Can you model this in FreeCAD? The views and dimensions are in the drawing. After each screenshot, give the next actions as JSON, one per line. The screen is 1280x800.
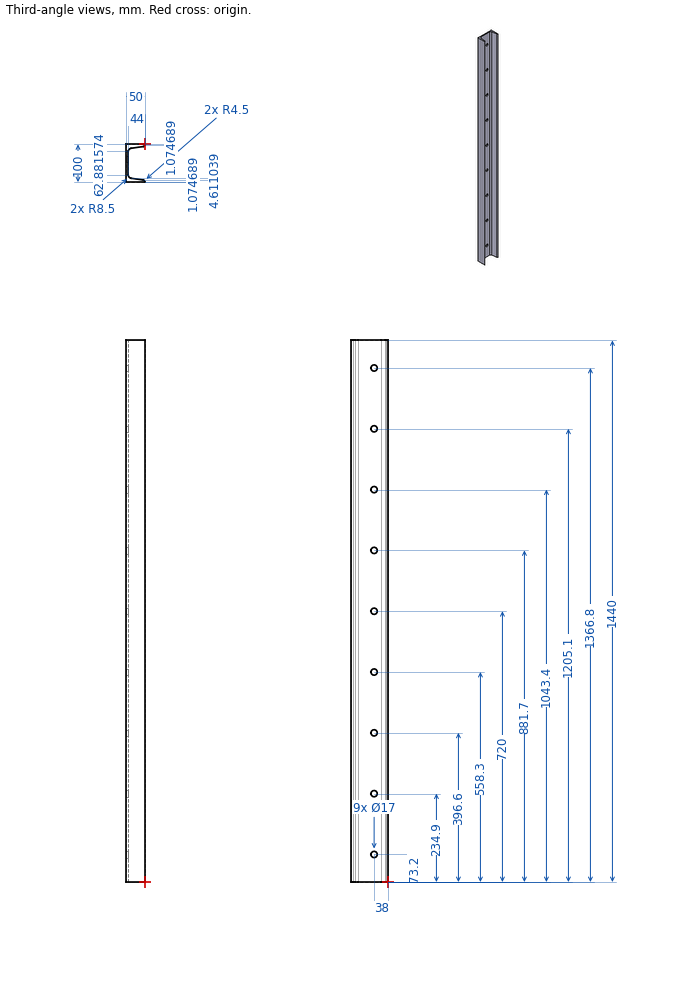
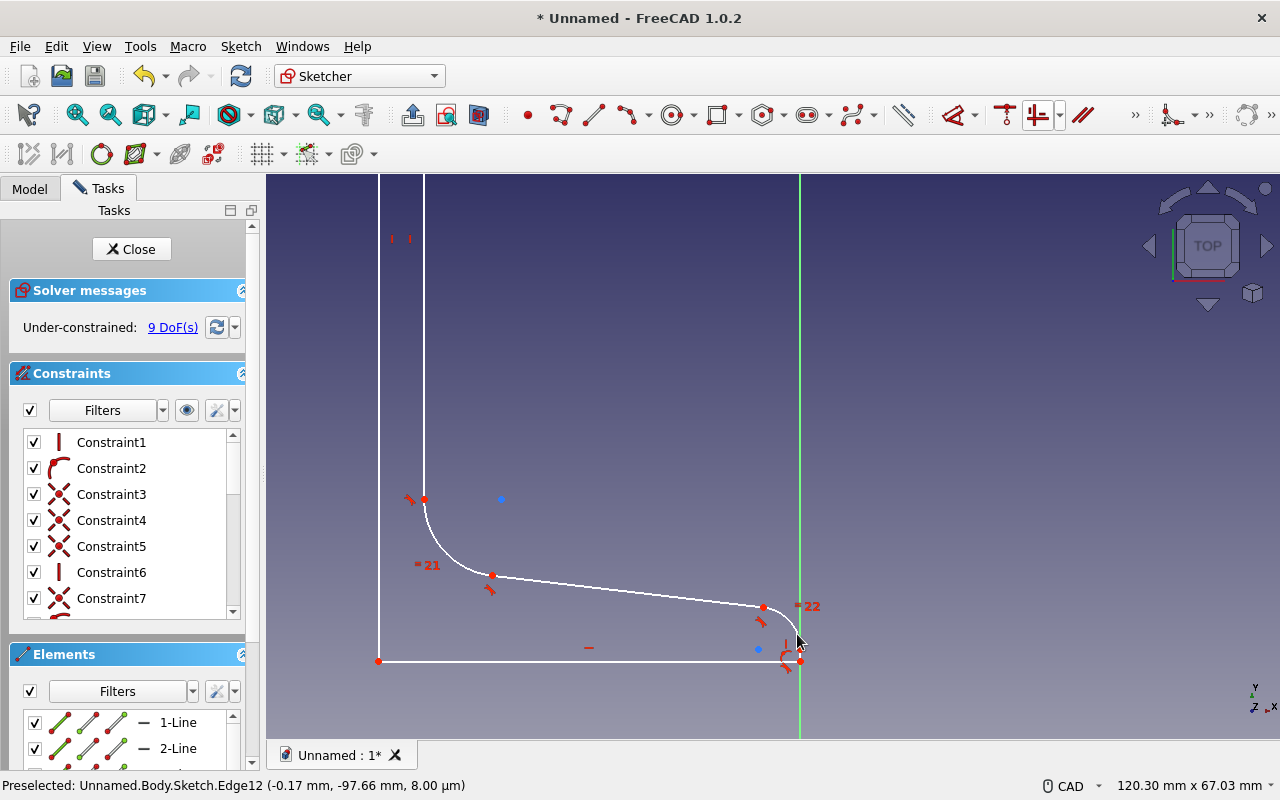
{"action": "left_click", "coordinate": [431, 532]}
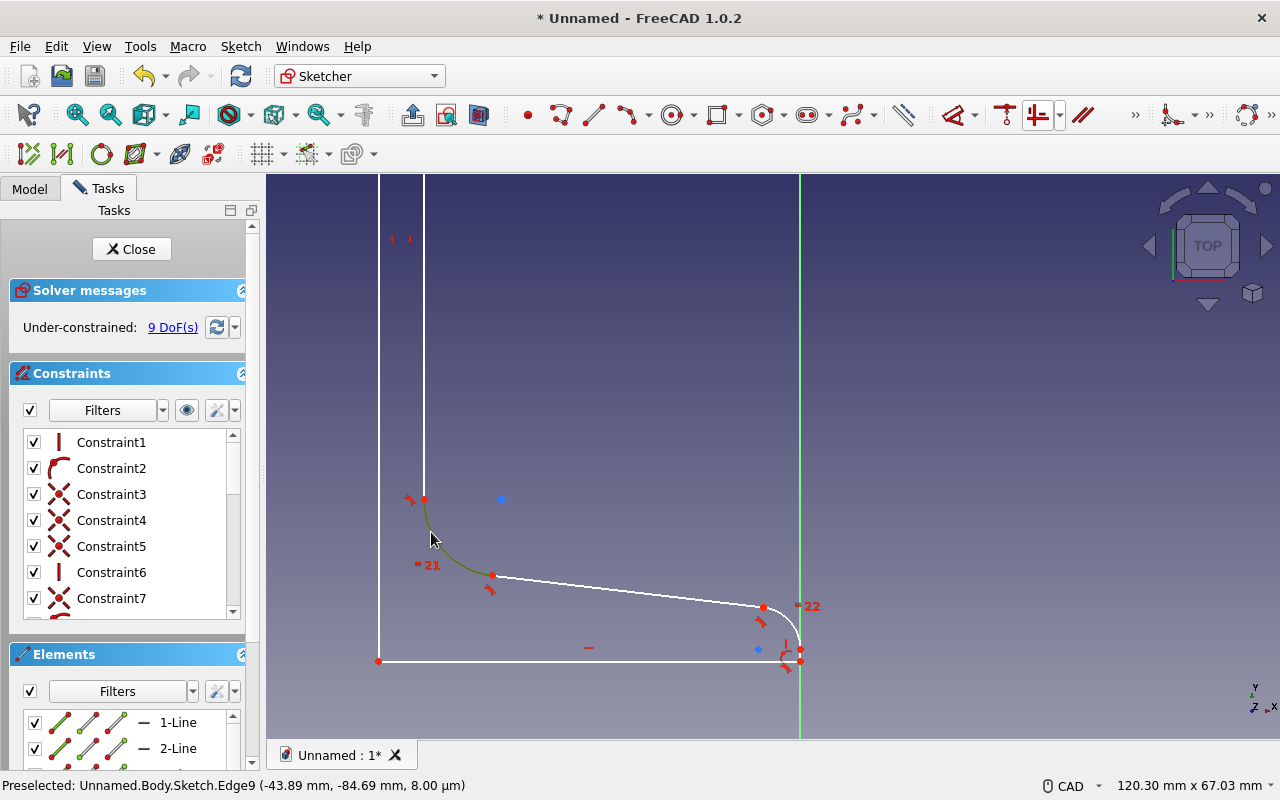
{"action": "left_click", "coordinate": [974, 116]}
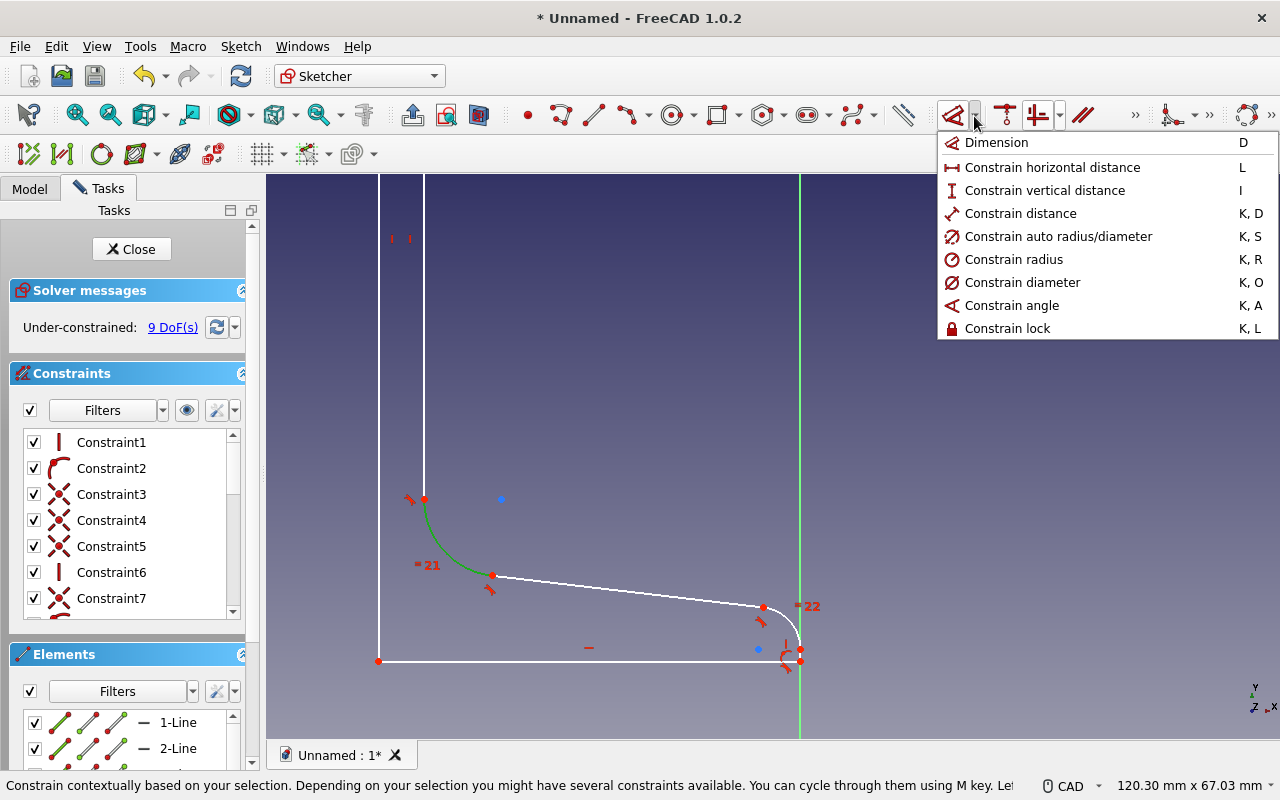
{"action": "left_click", "coordinate": [1108, 260]}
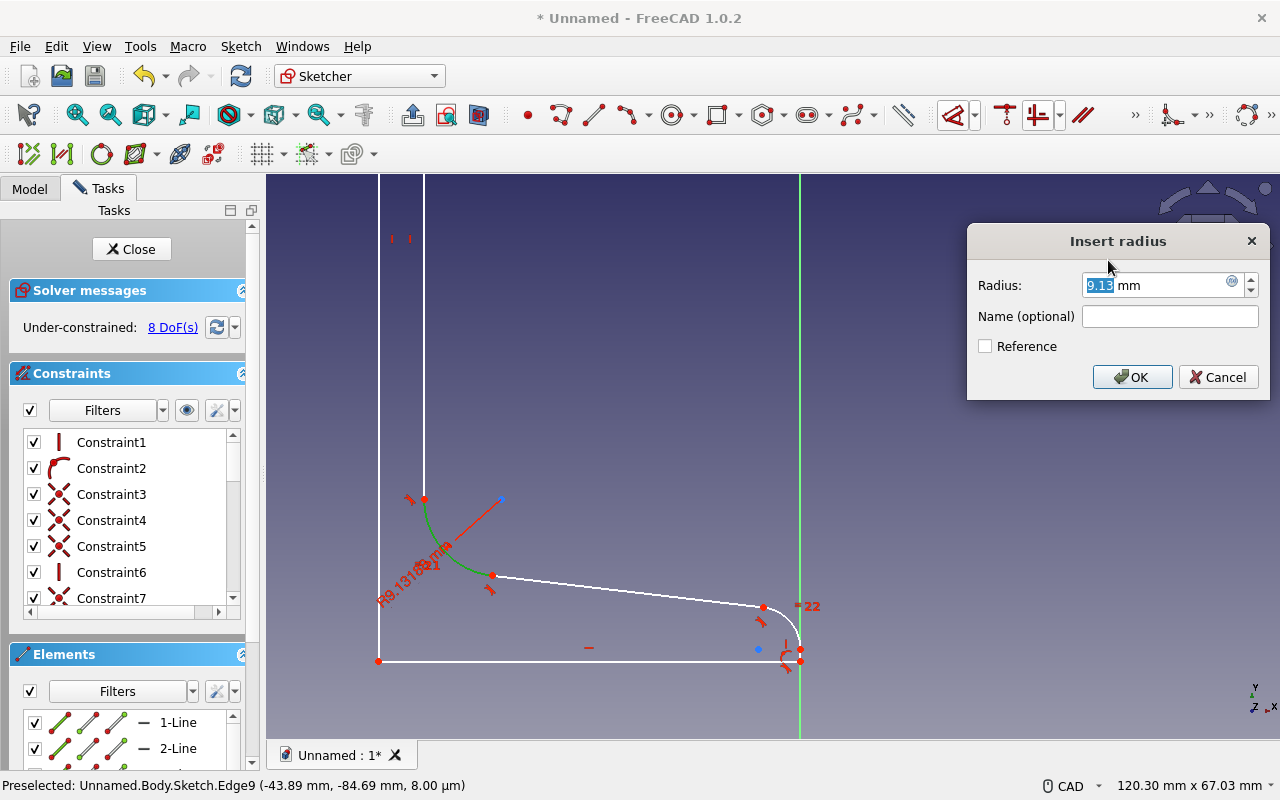
{"action": "type", "text": "8.5"}
{"action": "key", "text": "Return"}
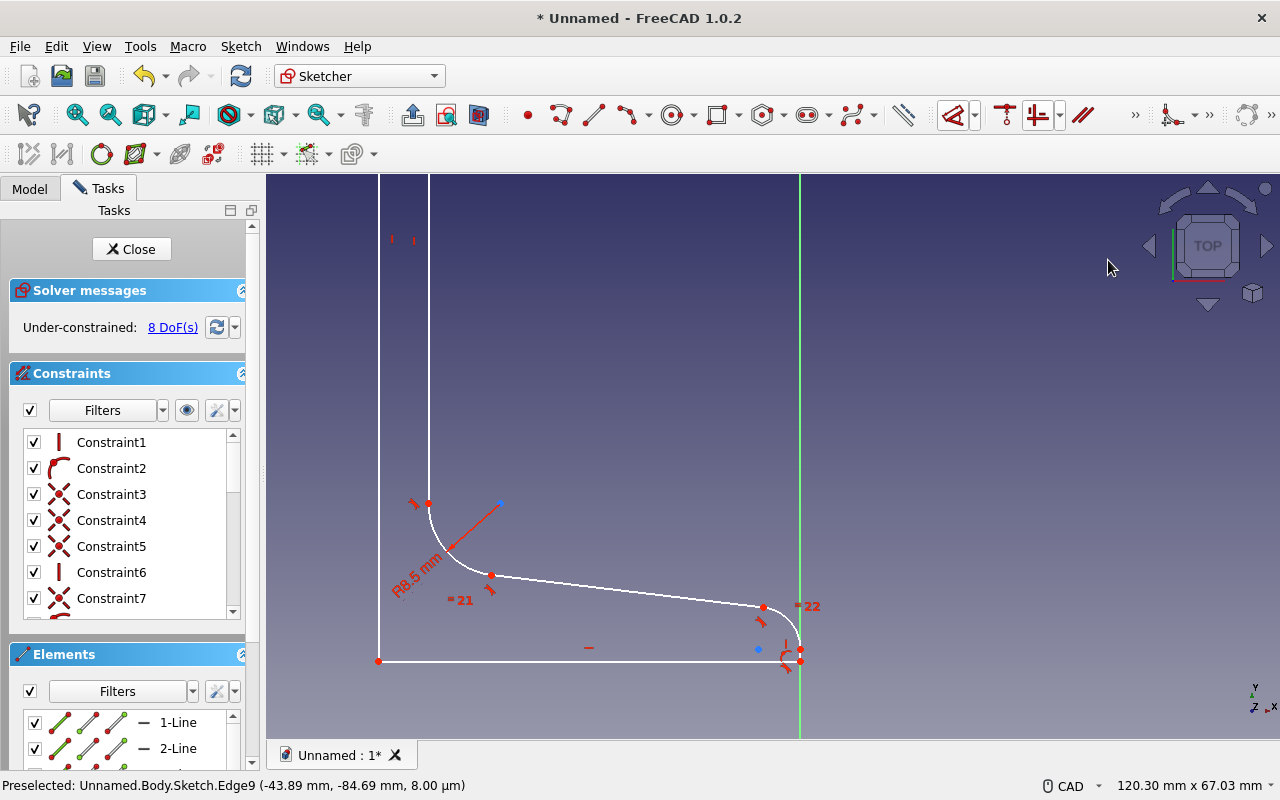
{"action": "scroll", "coordinate": [798, 635], "scroll_direction": "down", "scroll_amount": 4}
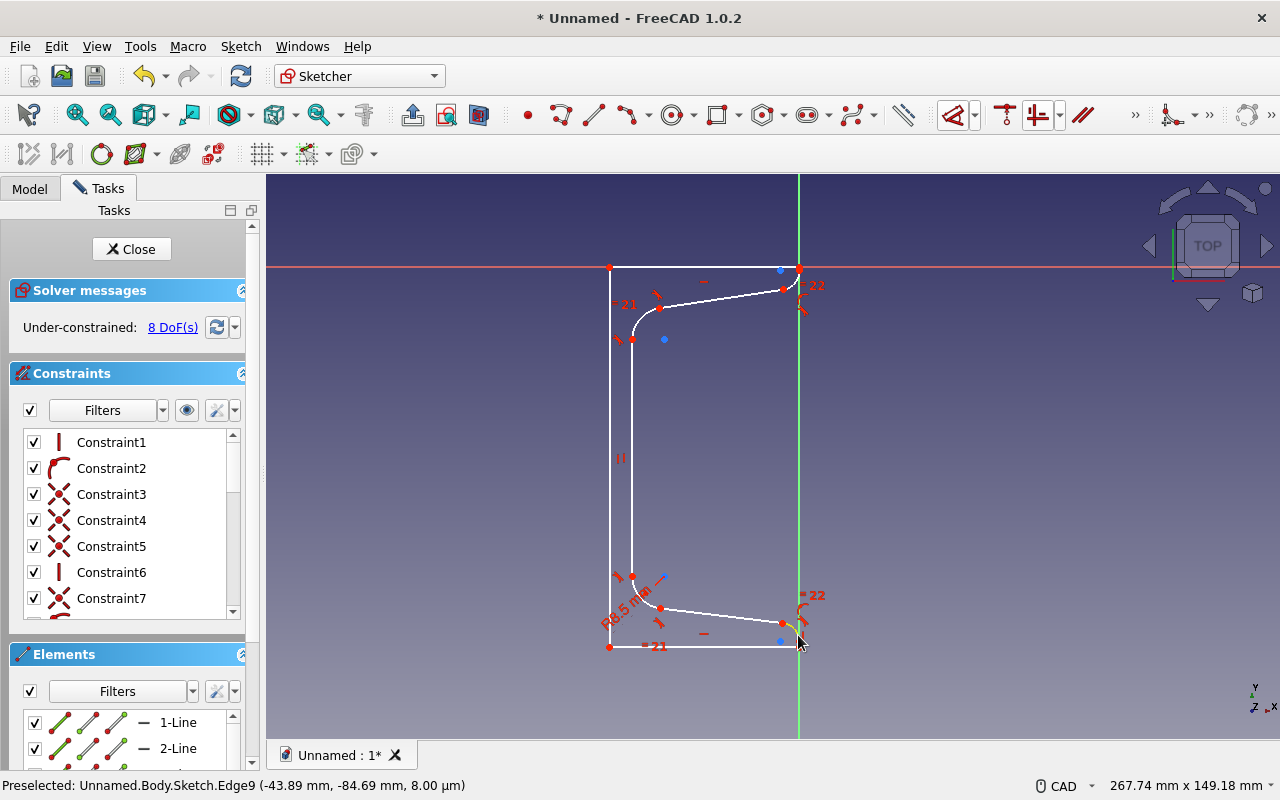
{"action": "scroll", "coordinate": [791, 287], "scroll_direction": "up", "scroll_amount": 5}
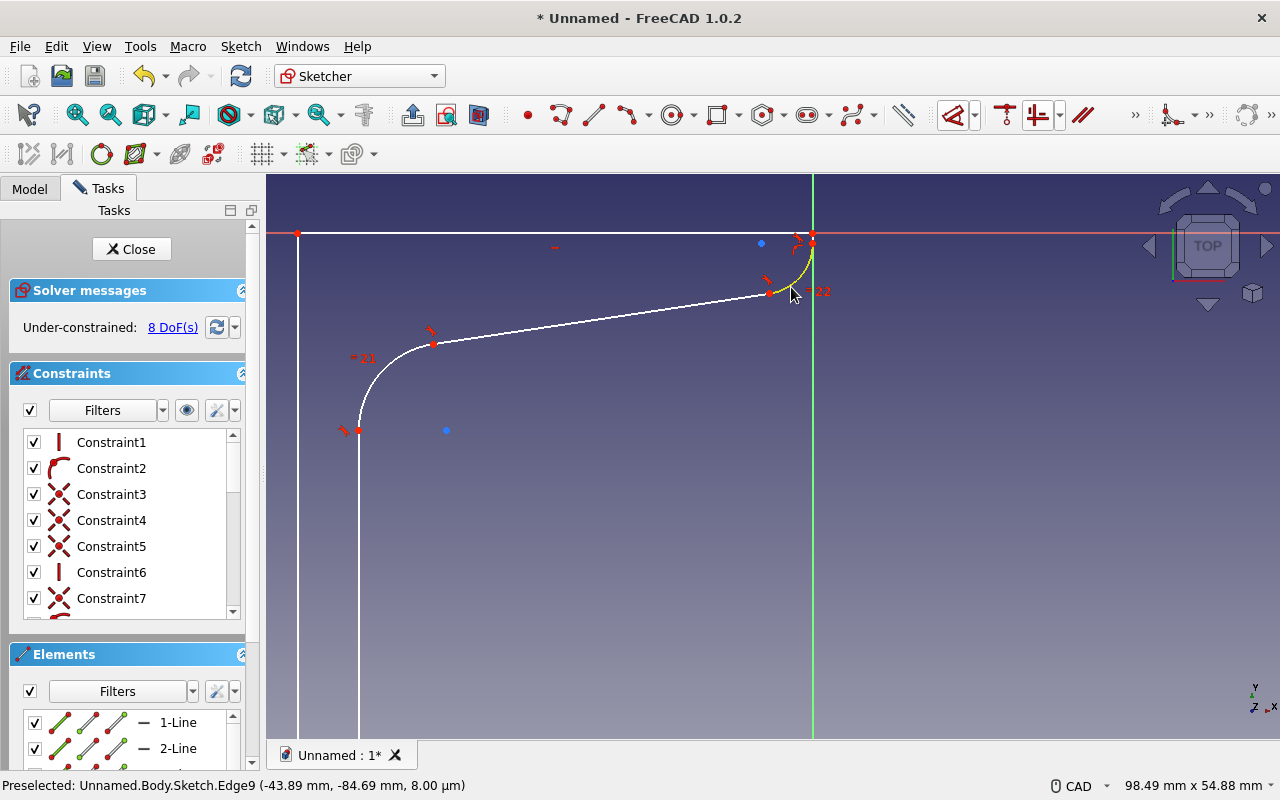
{"action": "left_click", "coordinate": [790, 286]}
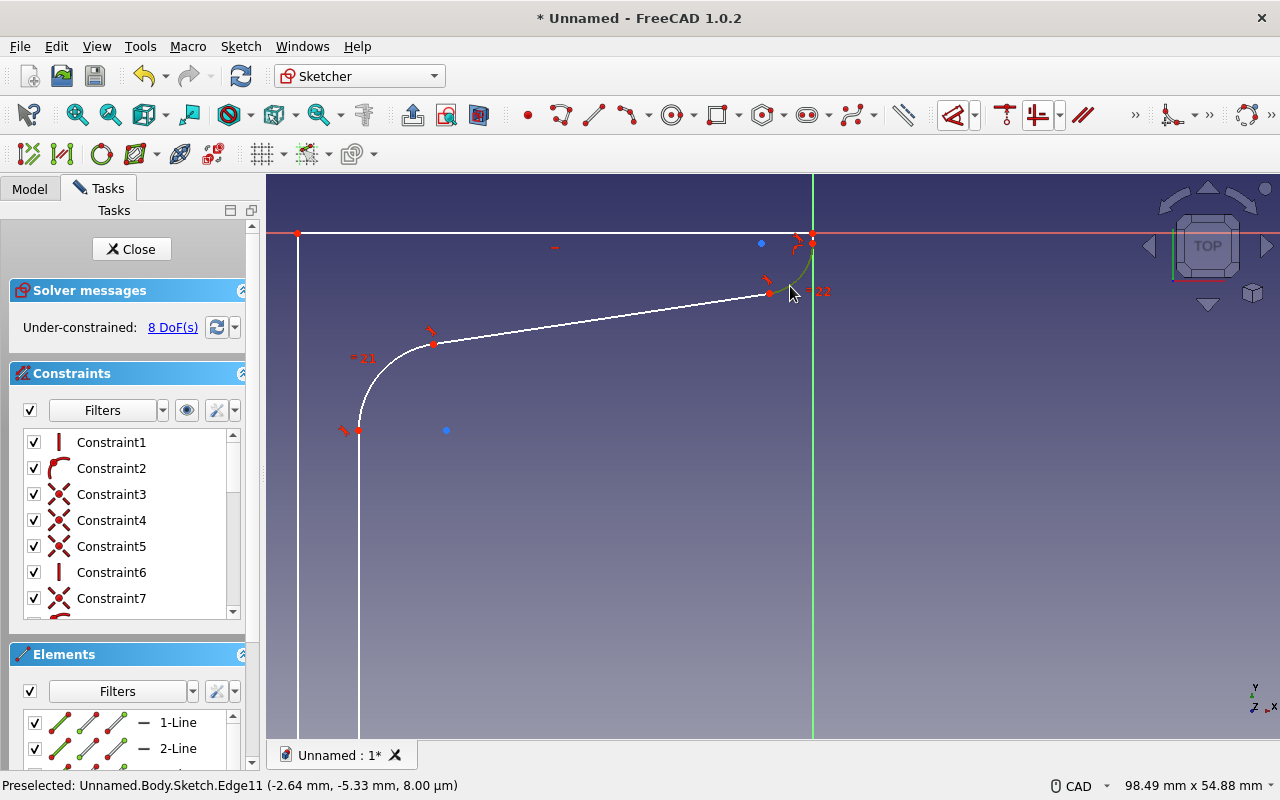
{"action": "key", "text": "k r"}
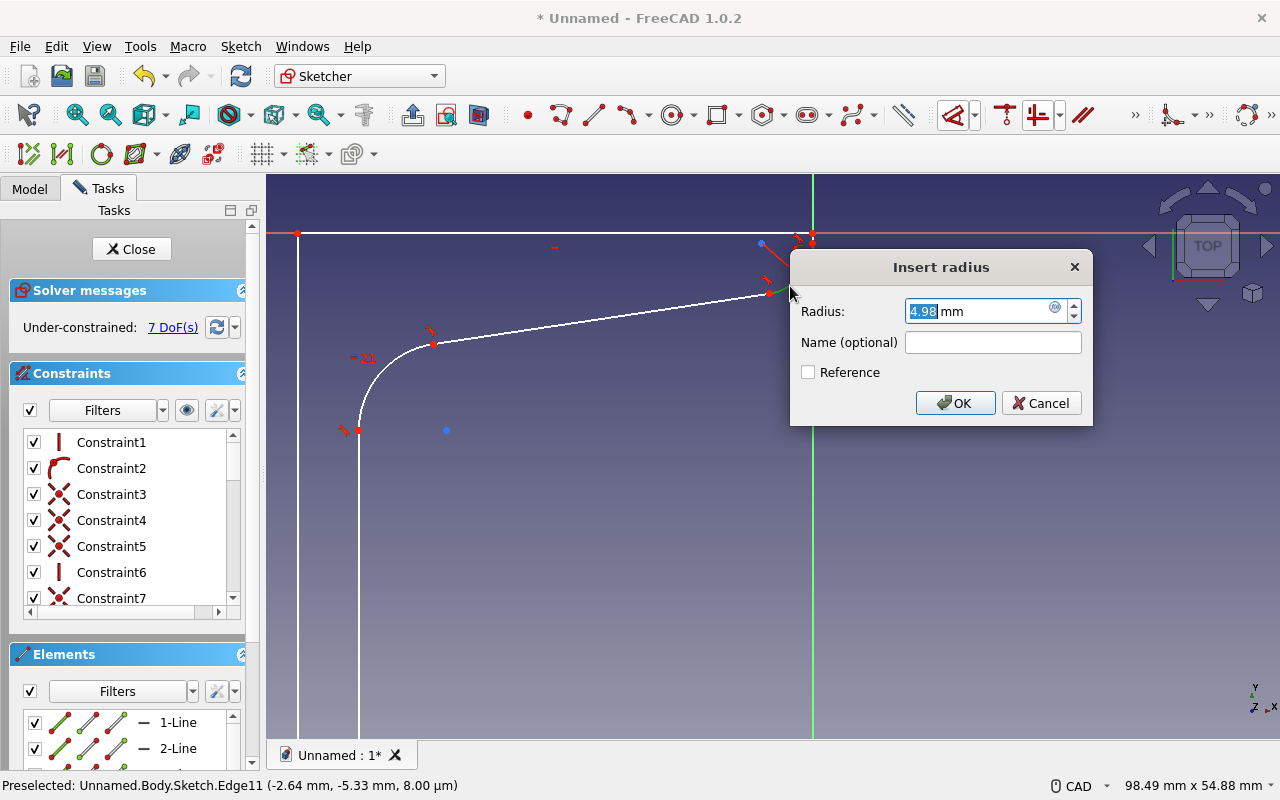
{"action": "type", "text": "4.5"}
{"action": "key", "text": "Return"}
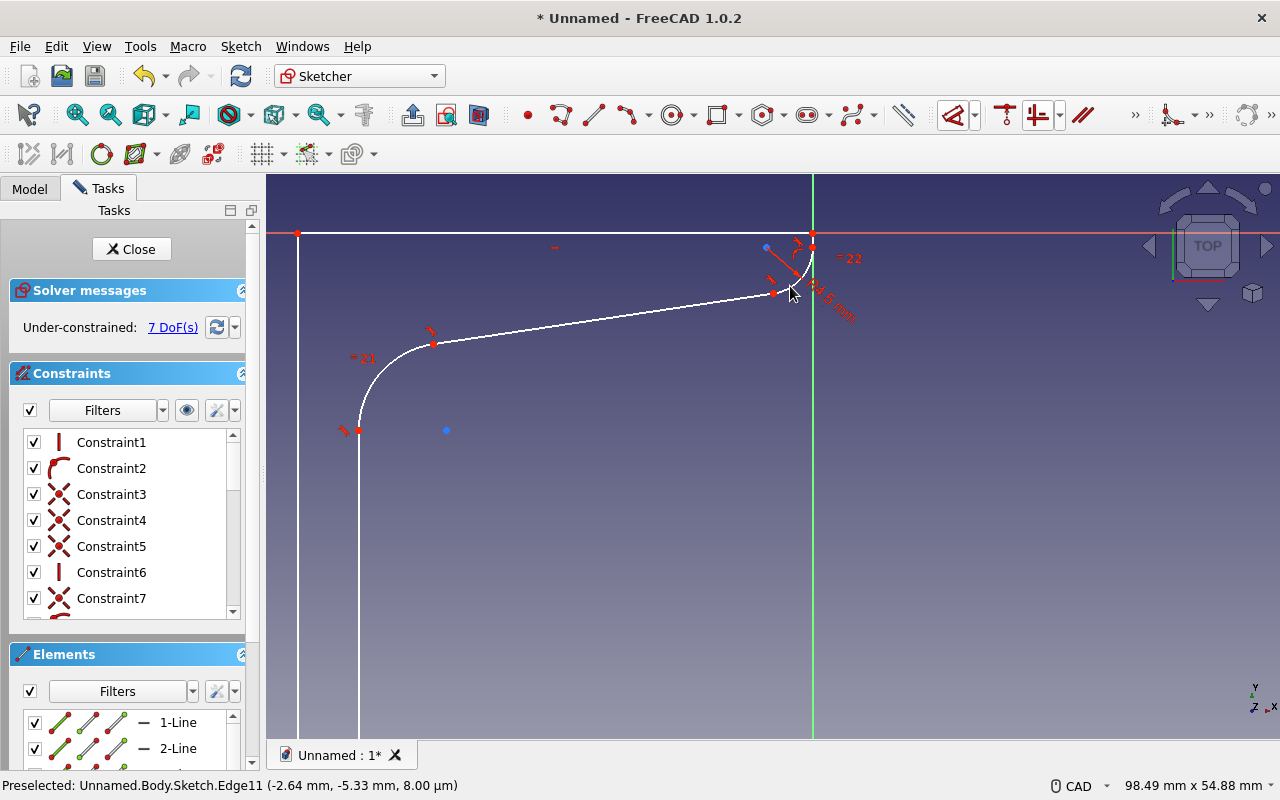
{"action": "left_click", "coordinate": [658, 233]}